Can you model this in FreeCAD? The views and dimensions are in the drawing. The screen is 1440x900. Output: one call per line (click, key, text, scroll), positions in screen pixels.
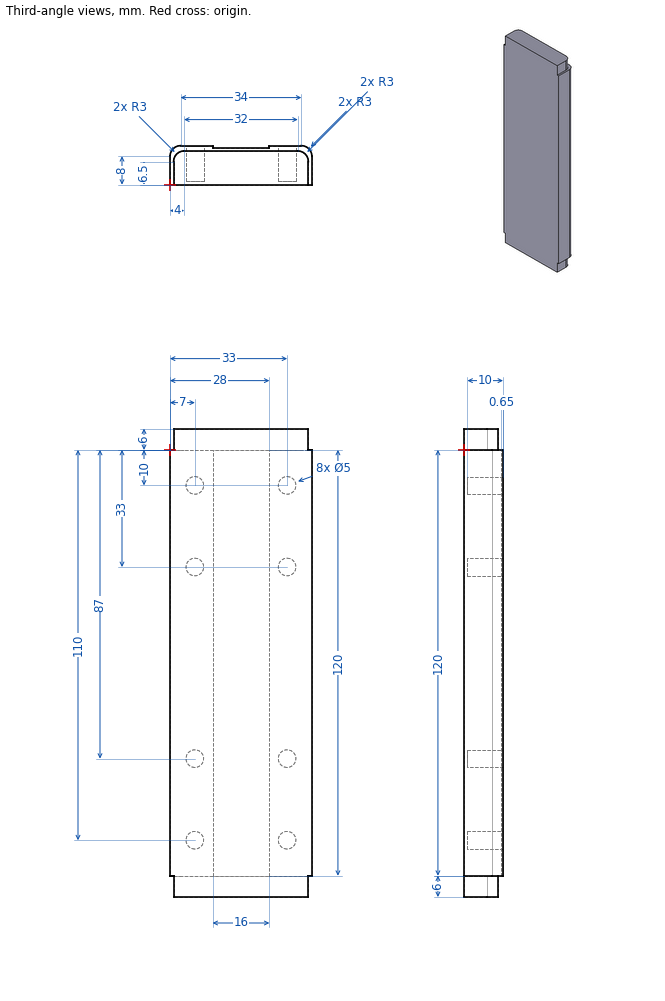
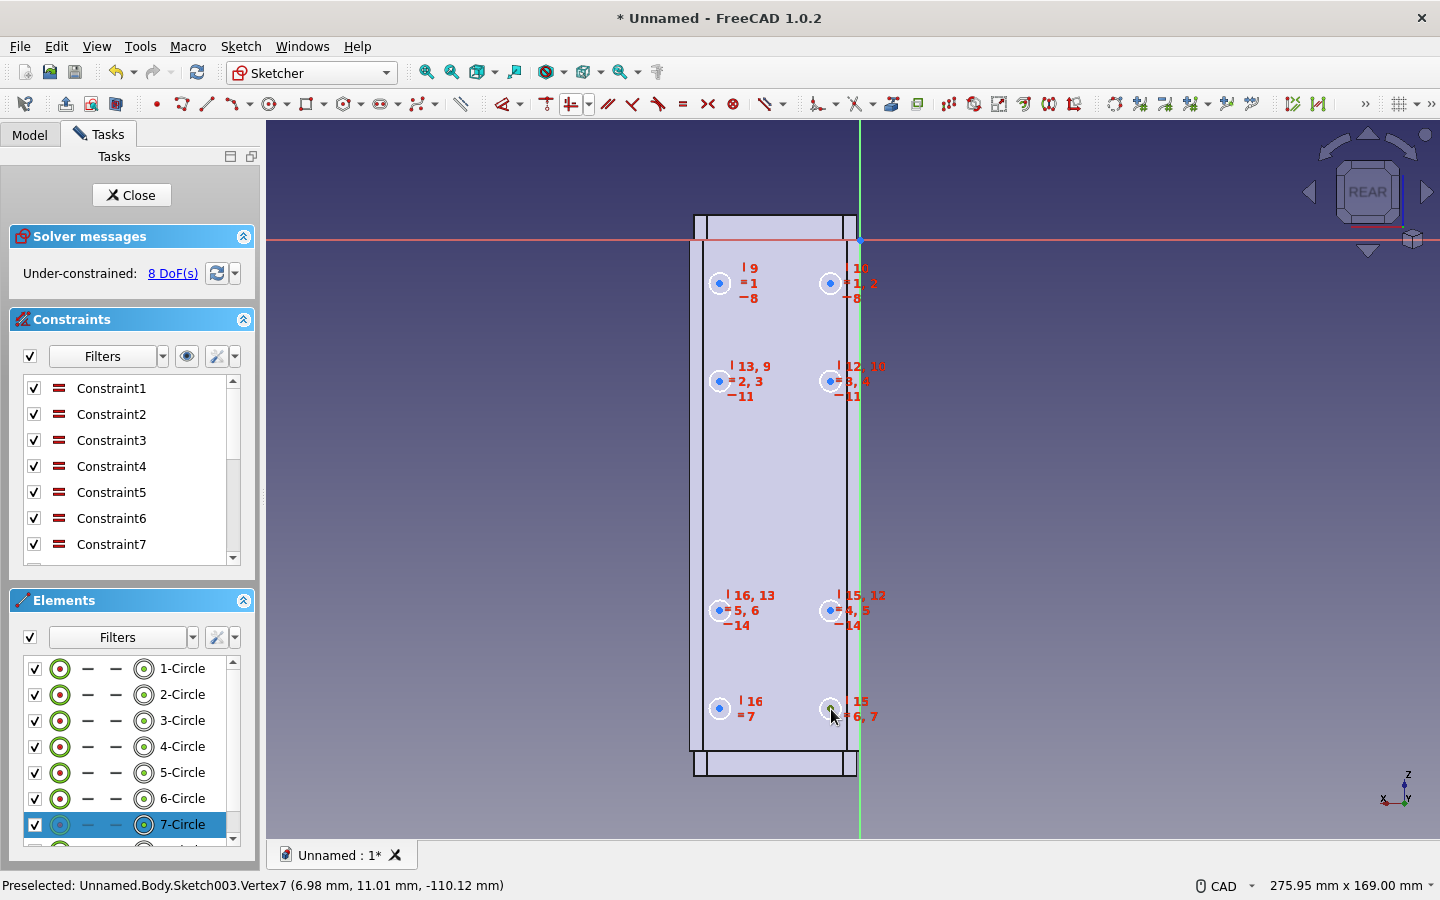
click(720, 709)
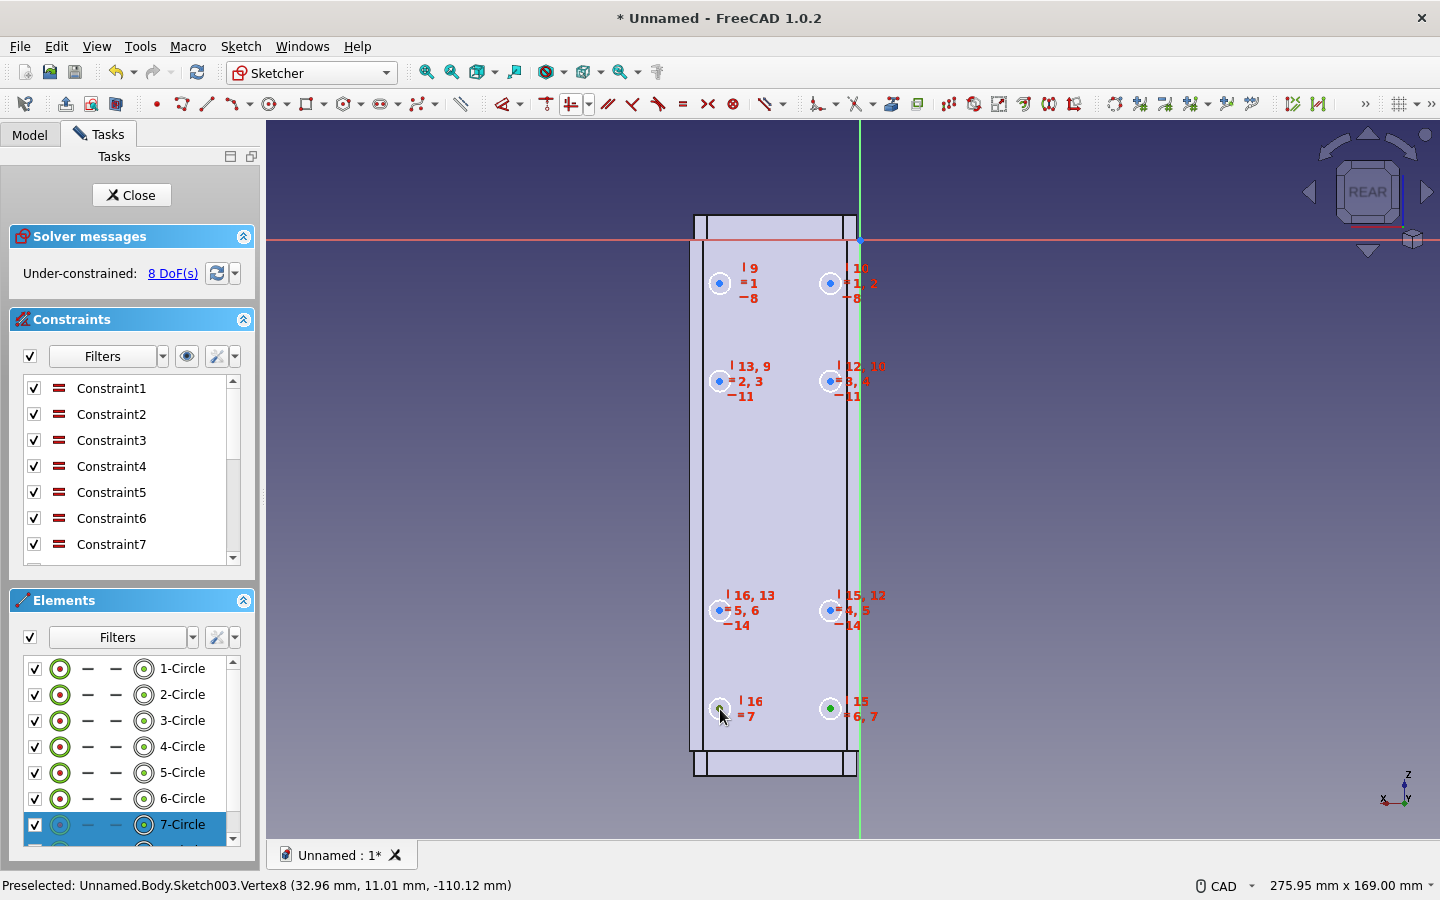
key(h)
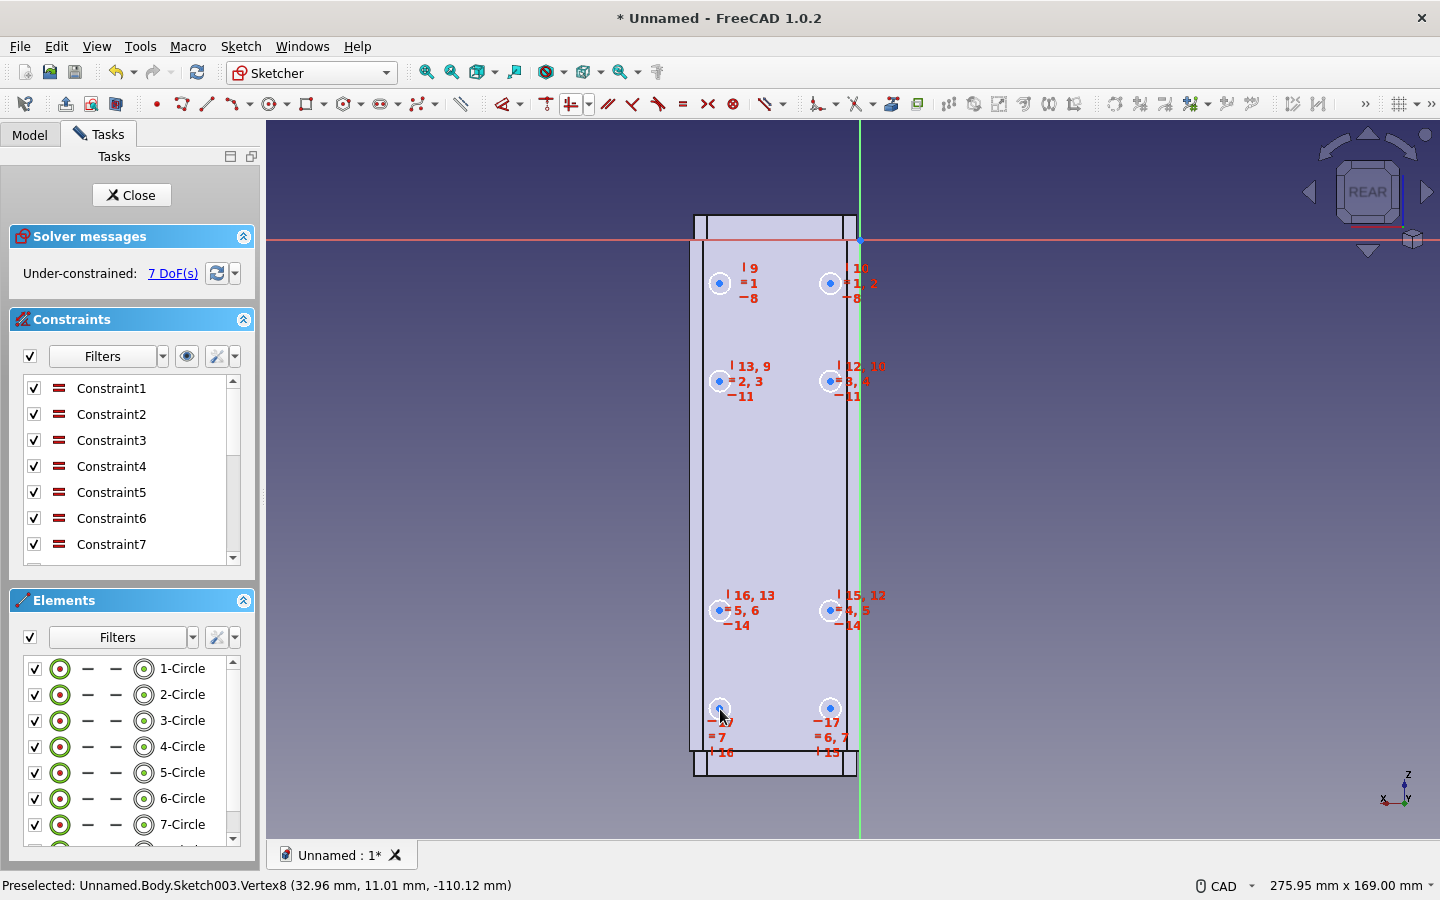
click(502, 104)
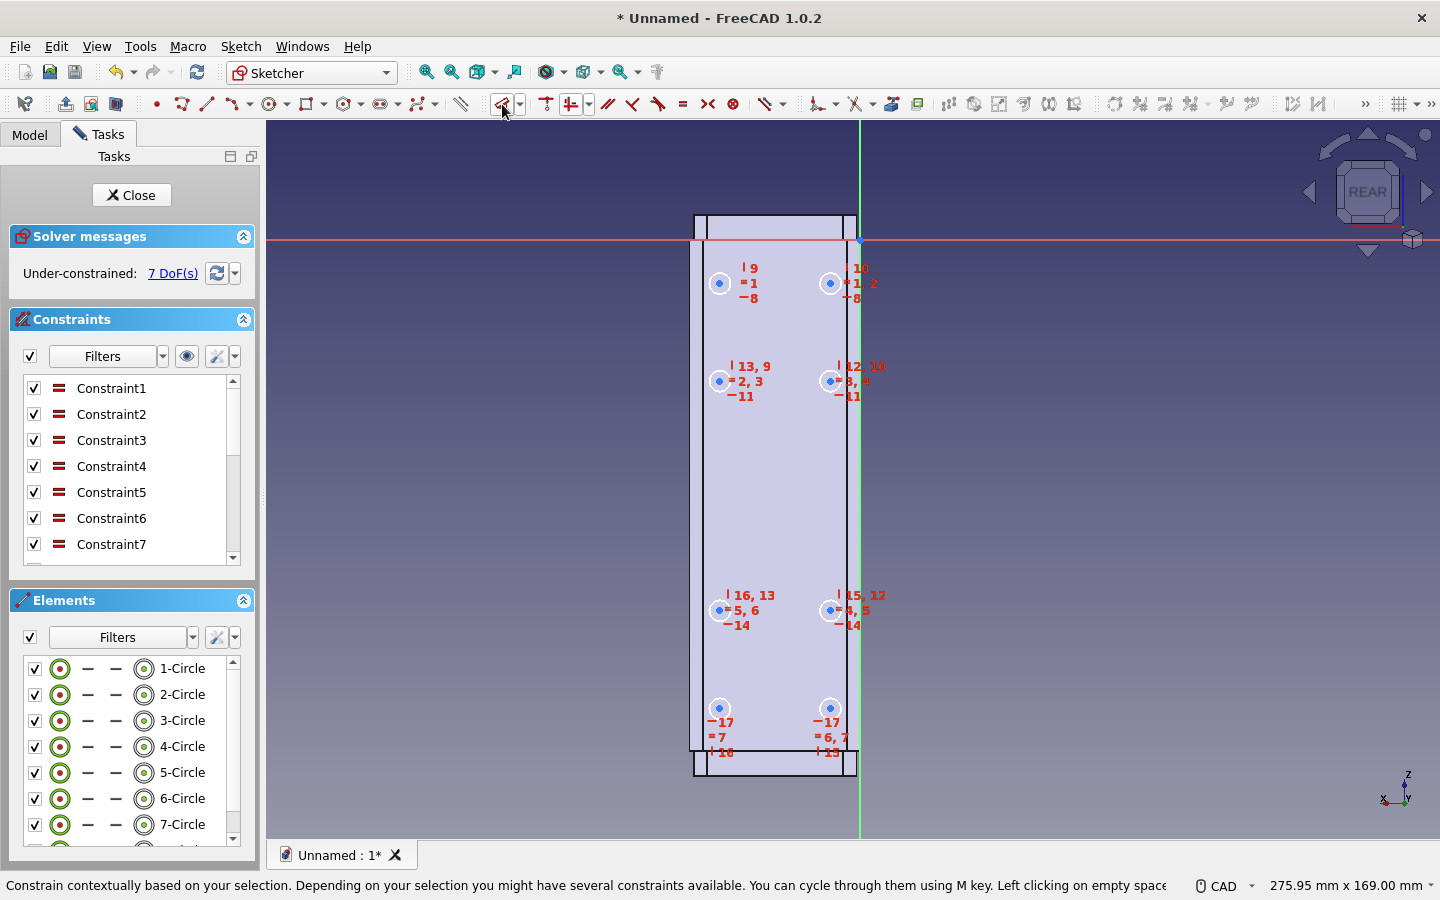
scroll(727, 276, up, 4)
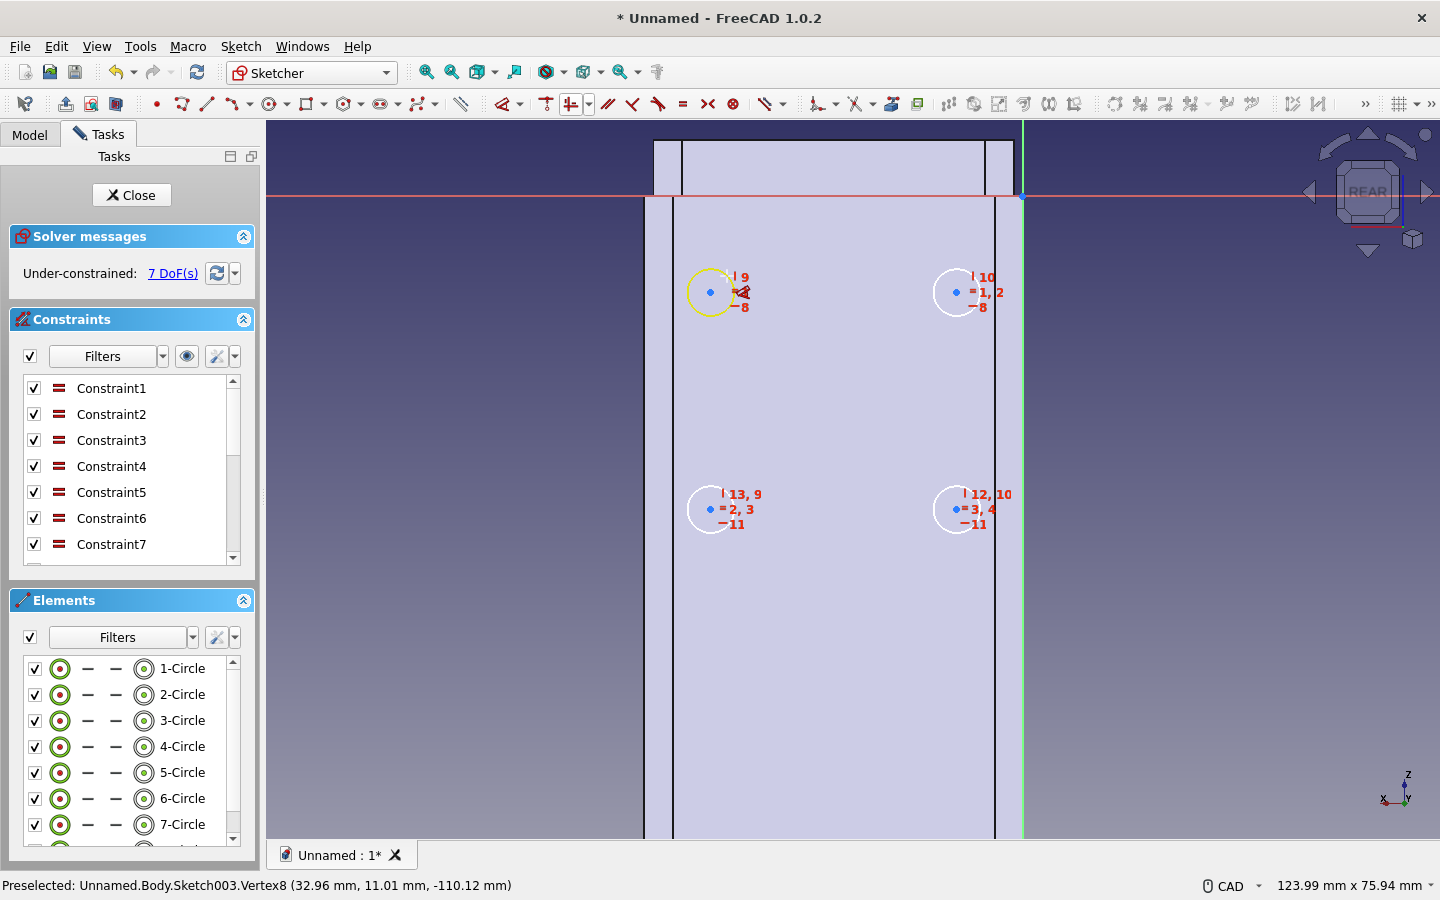
click(727, 276)
click(749, 253)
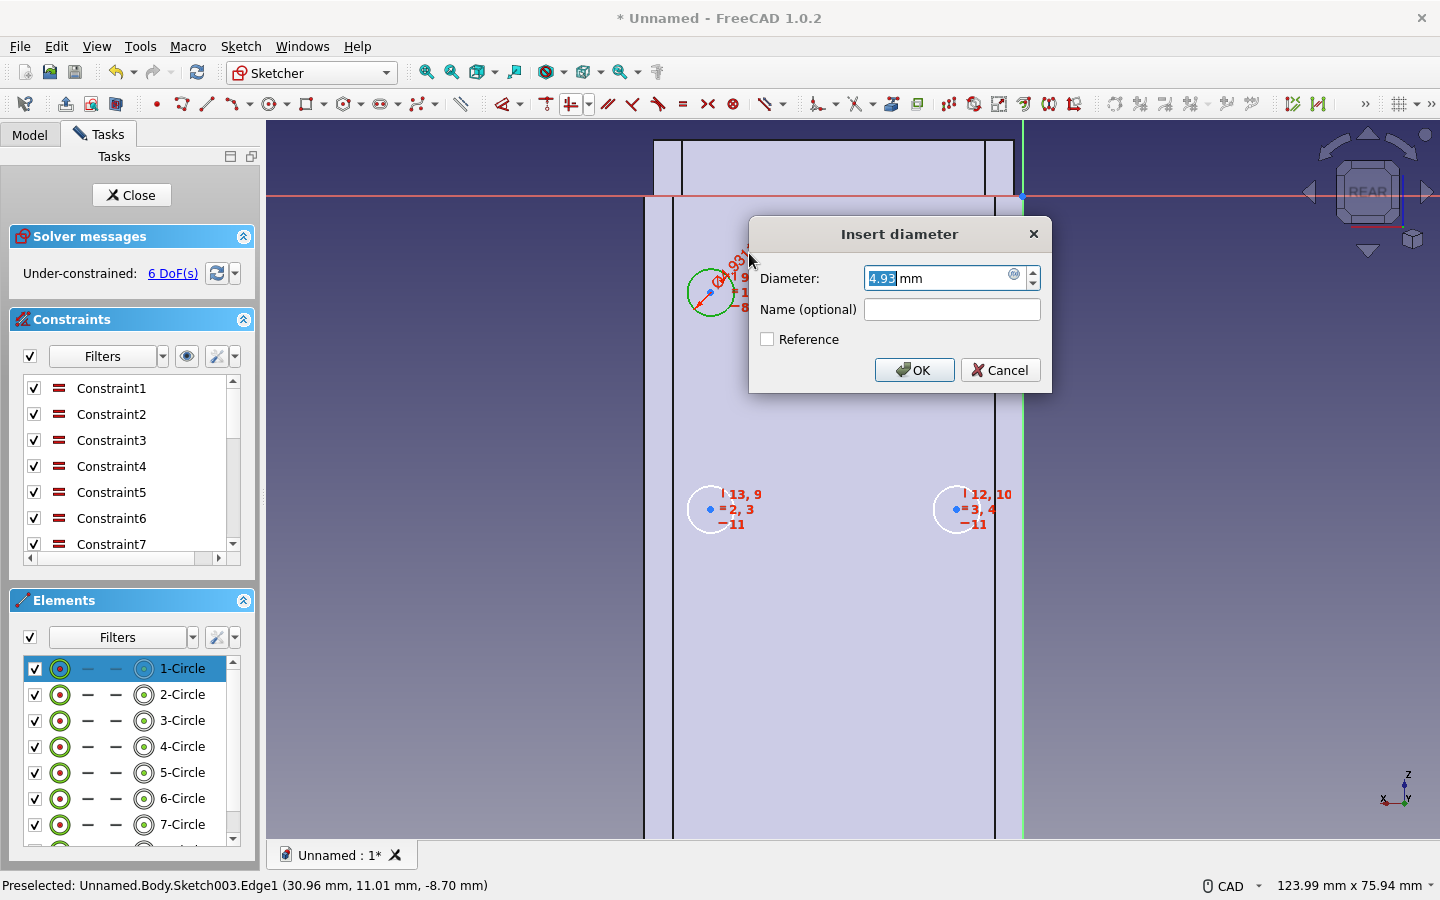
text(5)
key(Return)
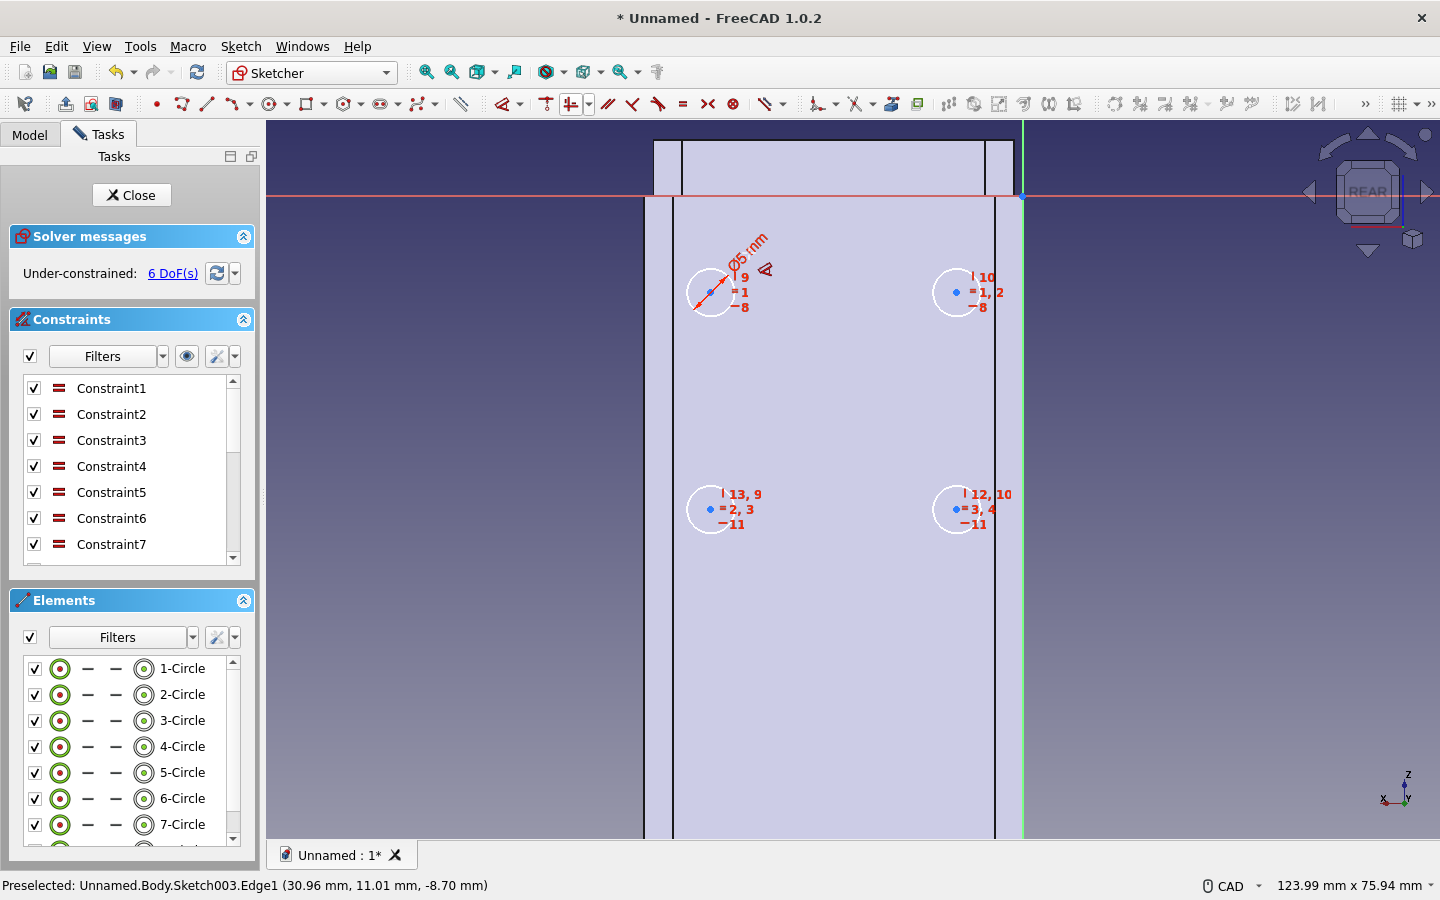
click(957, 293)
click(990, 162)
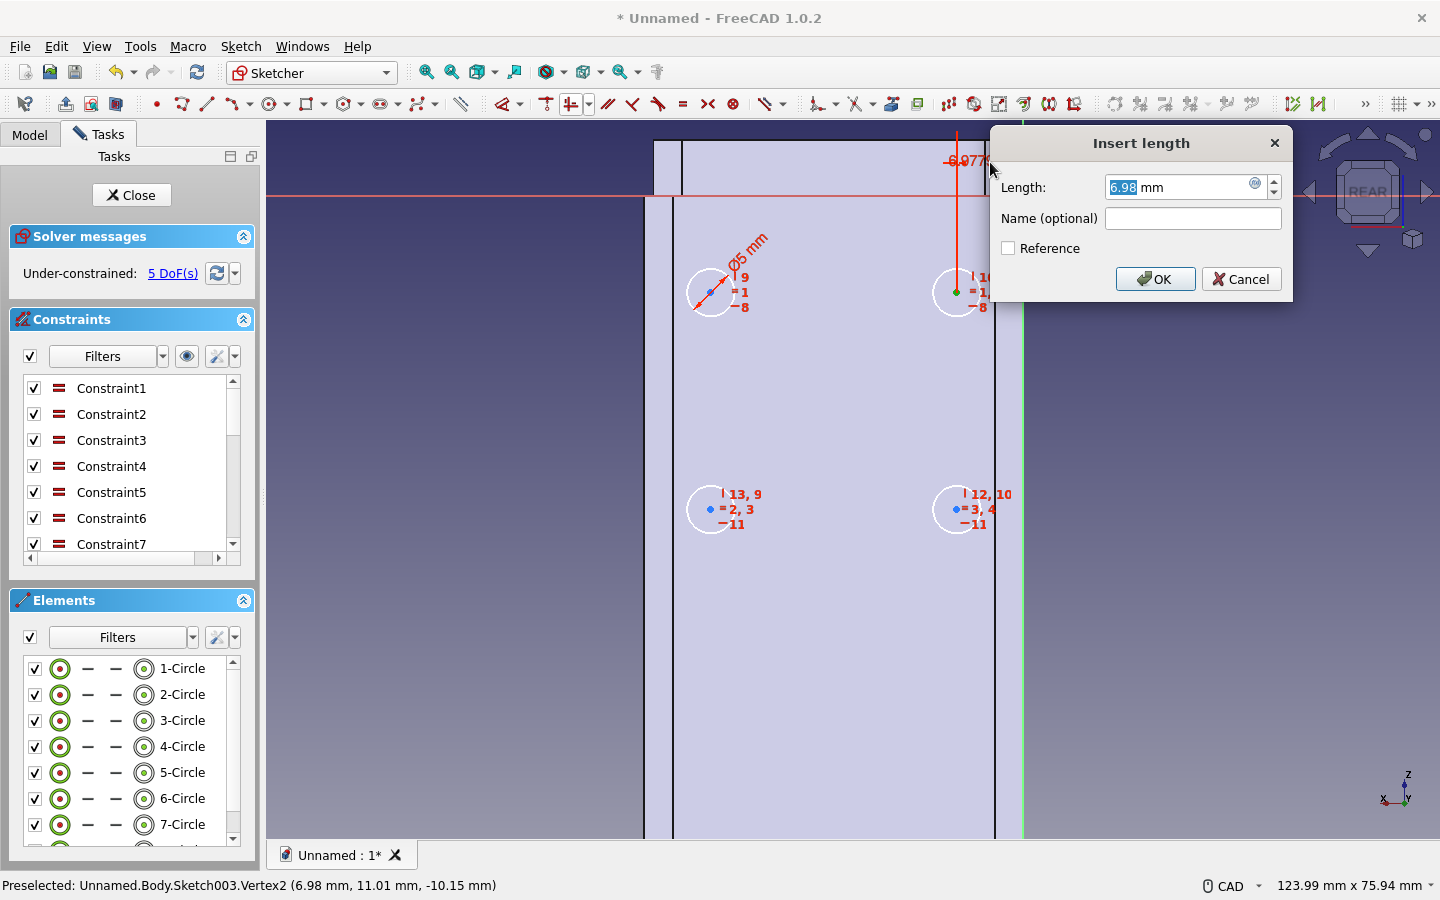
text(7)
key(Return)